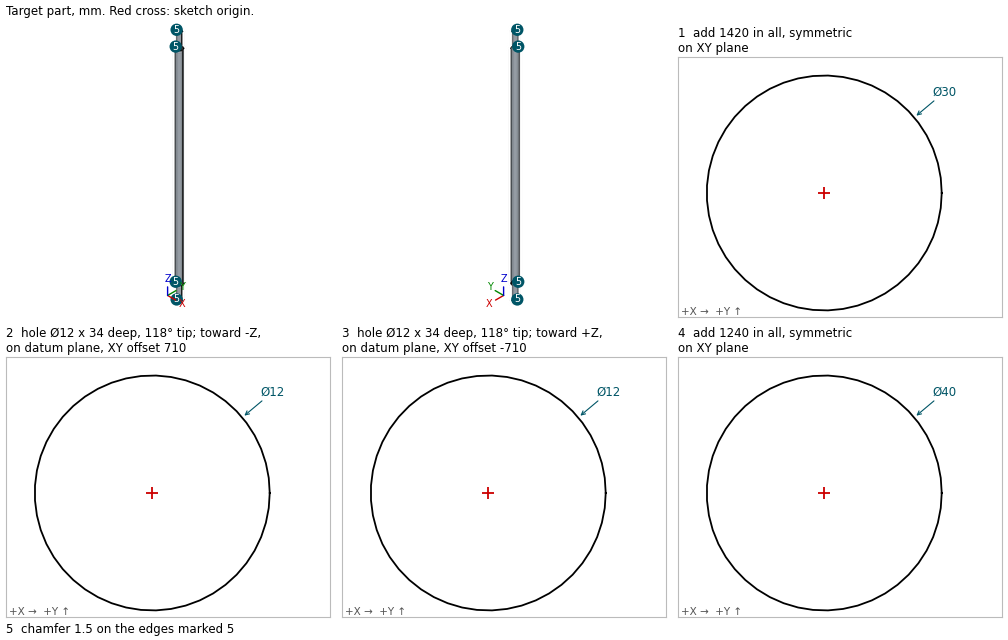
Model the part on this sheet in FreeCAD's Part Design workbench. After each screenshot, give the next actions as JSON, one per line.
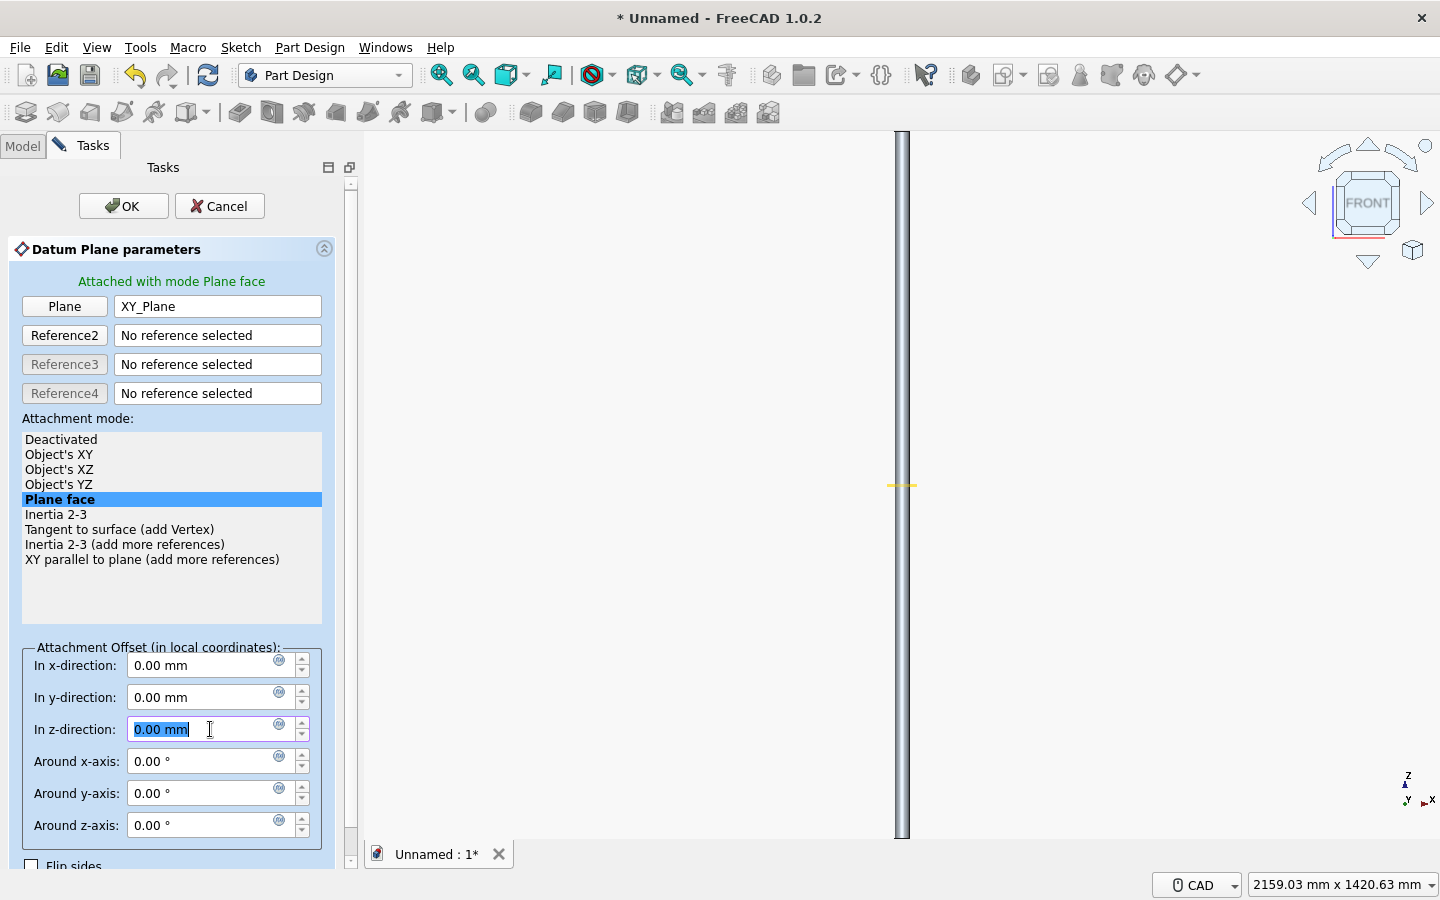
{"action": "type", "text": "710"}
{"action": "key", "text": "Tab"}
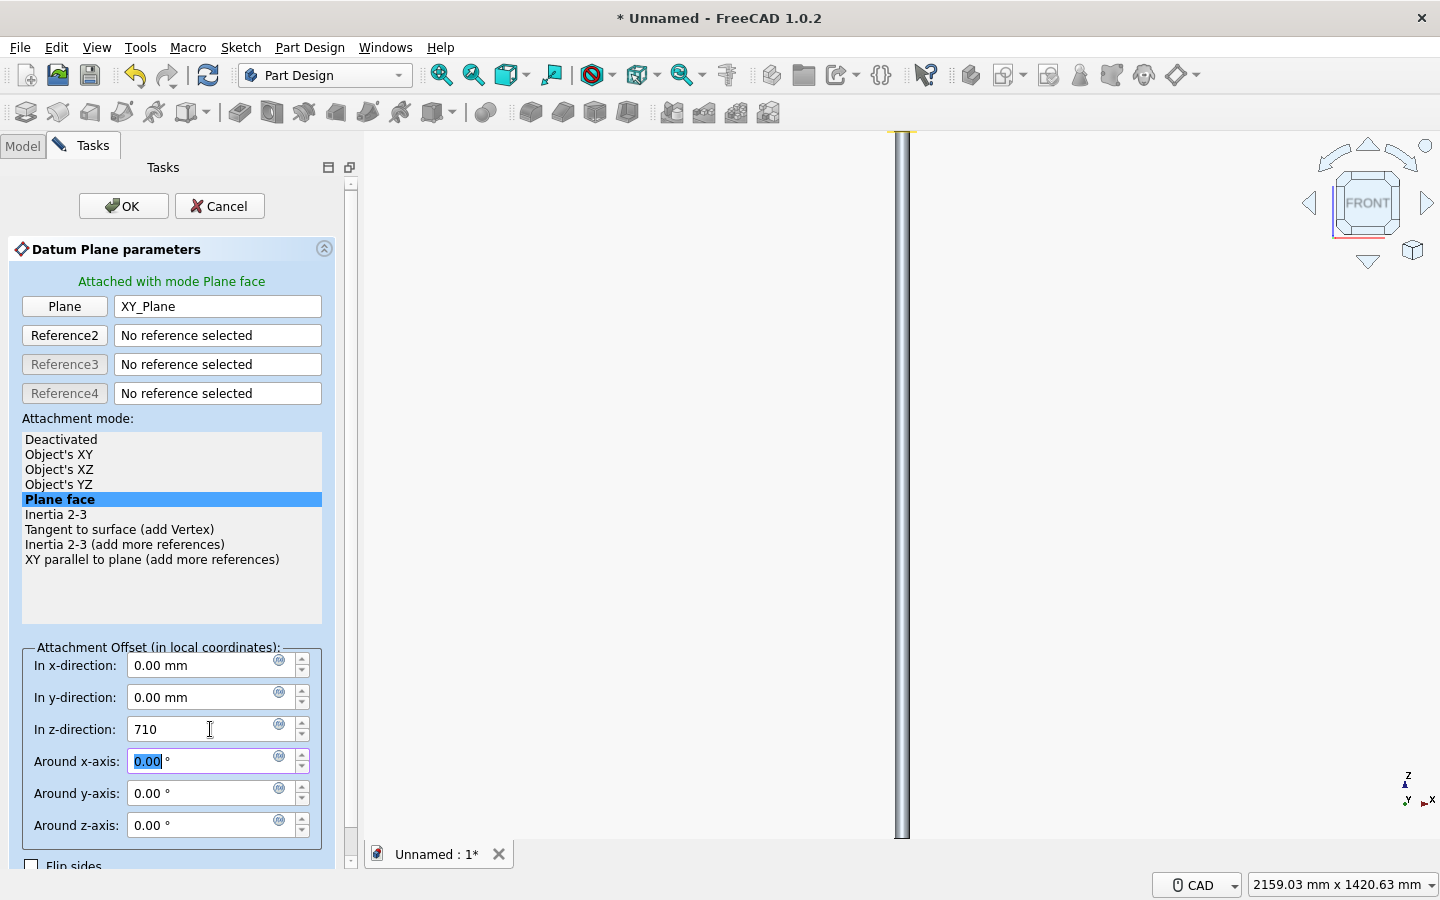
{"action": "left_click", "coordinate": [124, 206]}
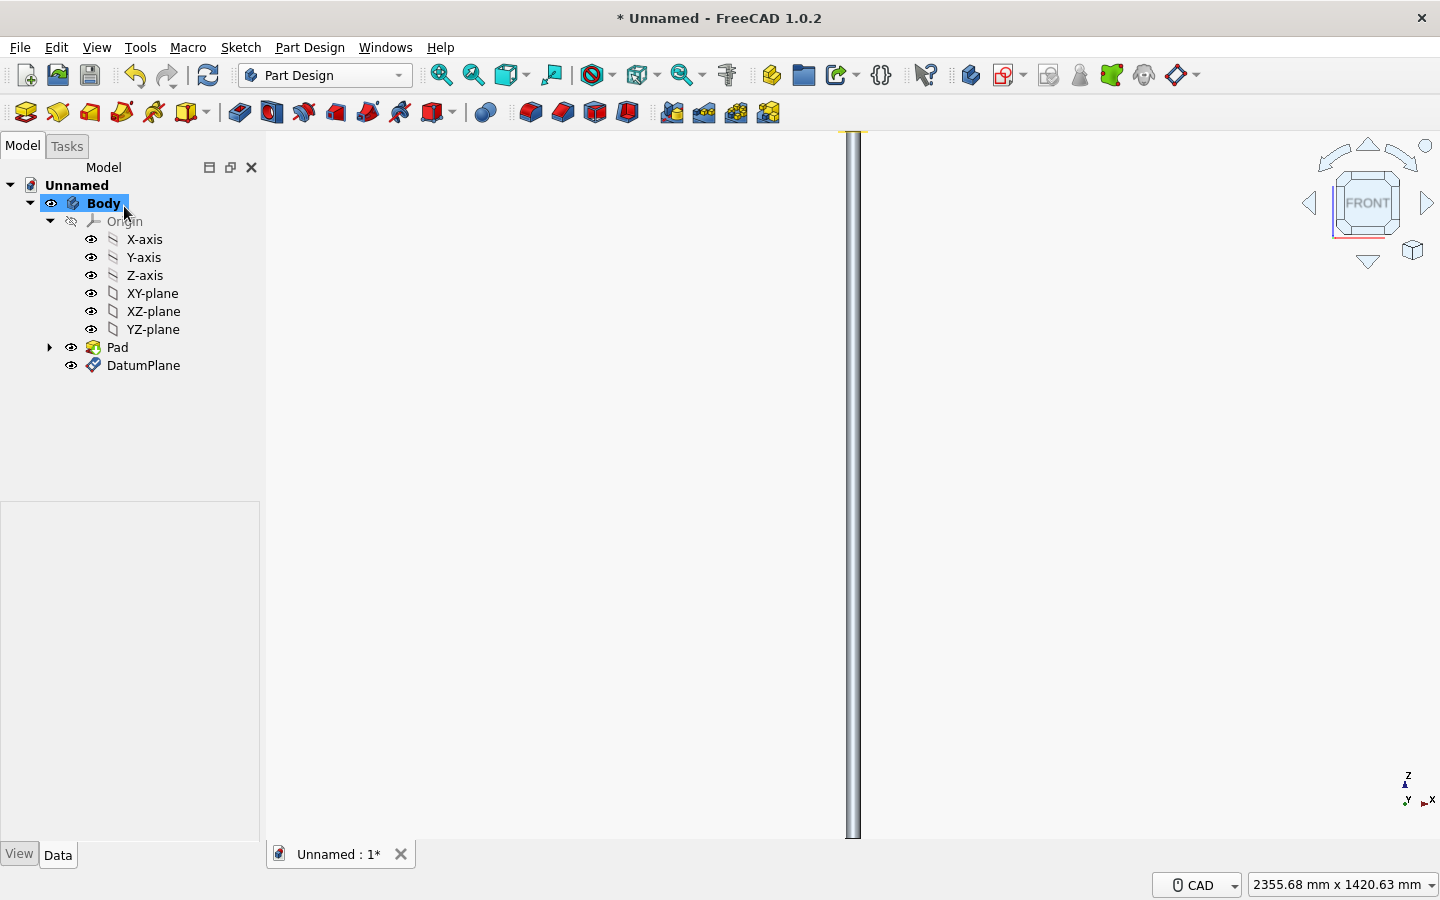
{"action": "left_click", "coordinate": [116, 365]}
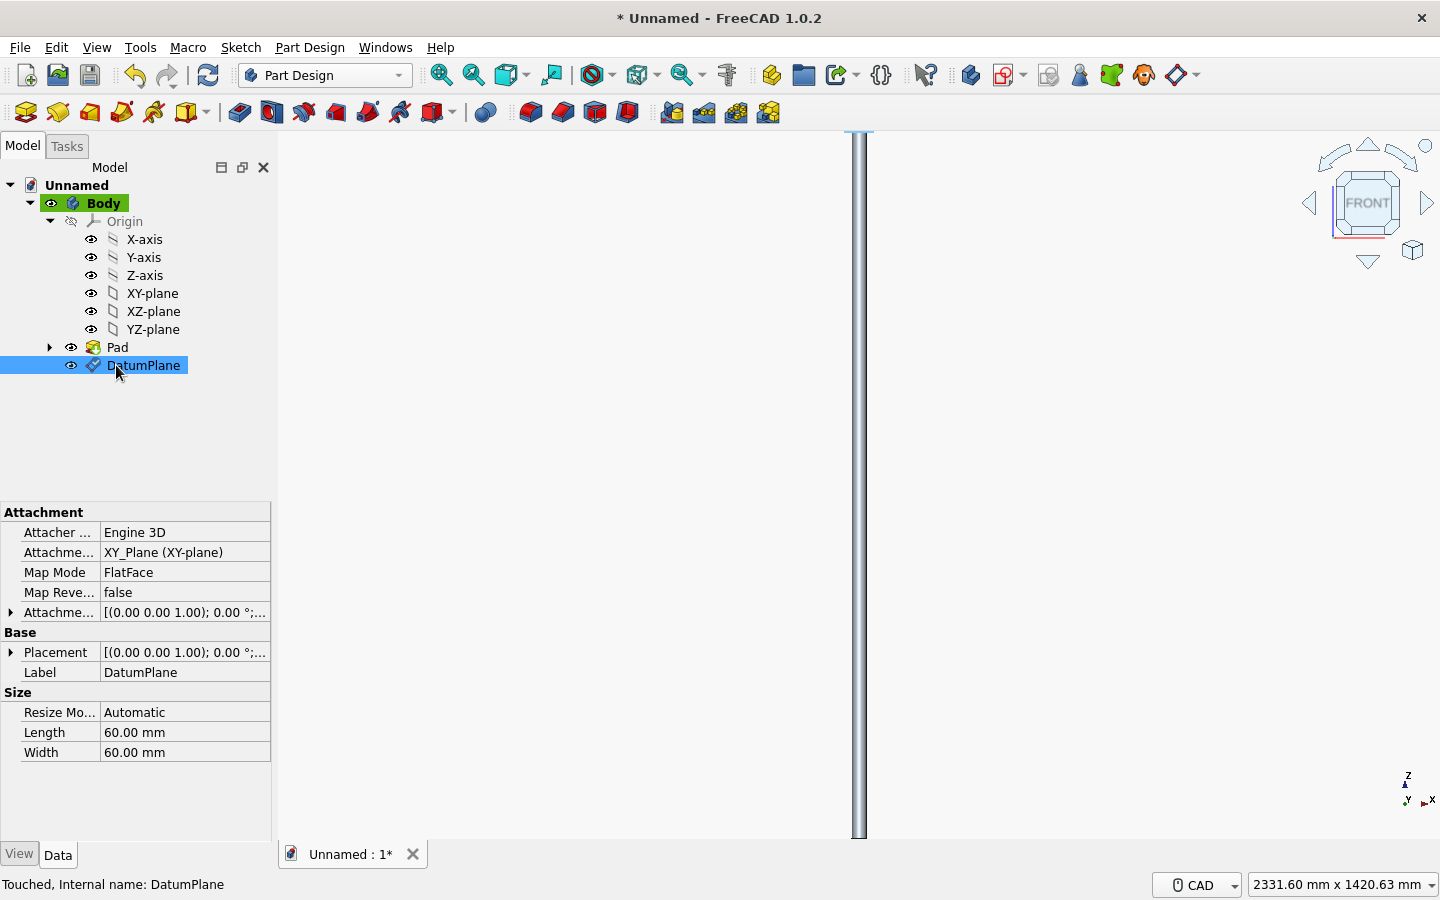
{"action": "left_click", "coordinate": [1004, 76]}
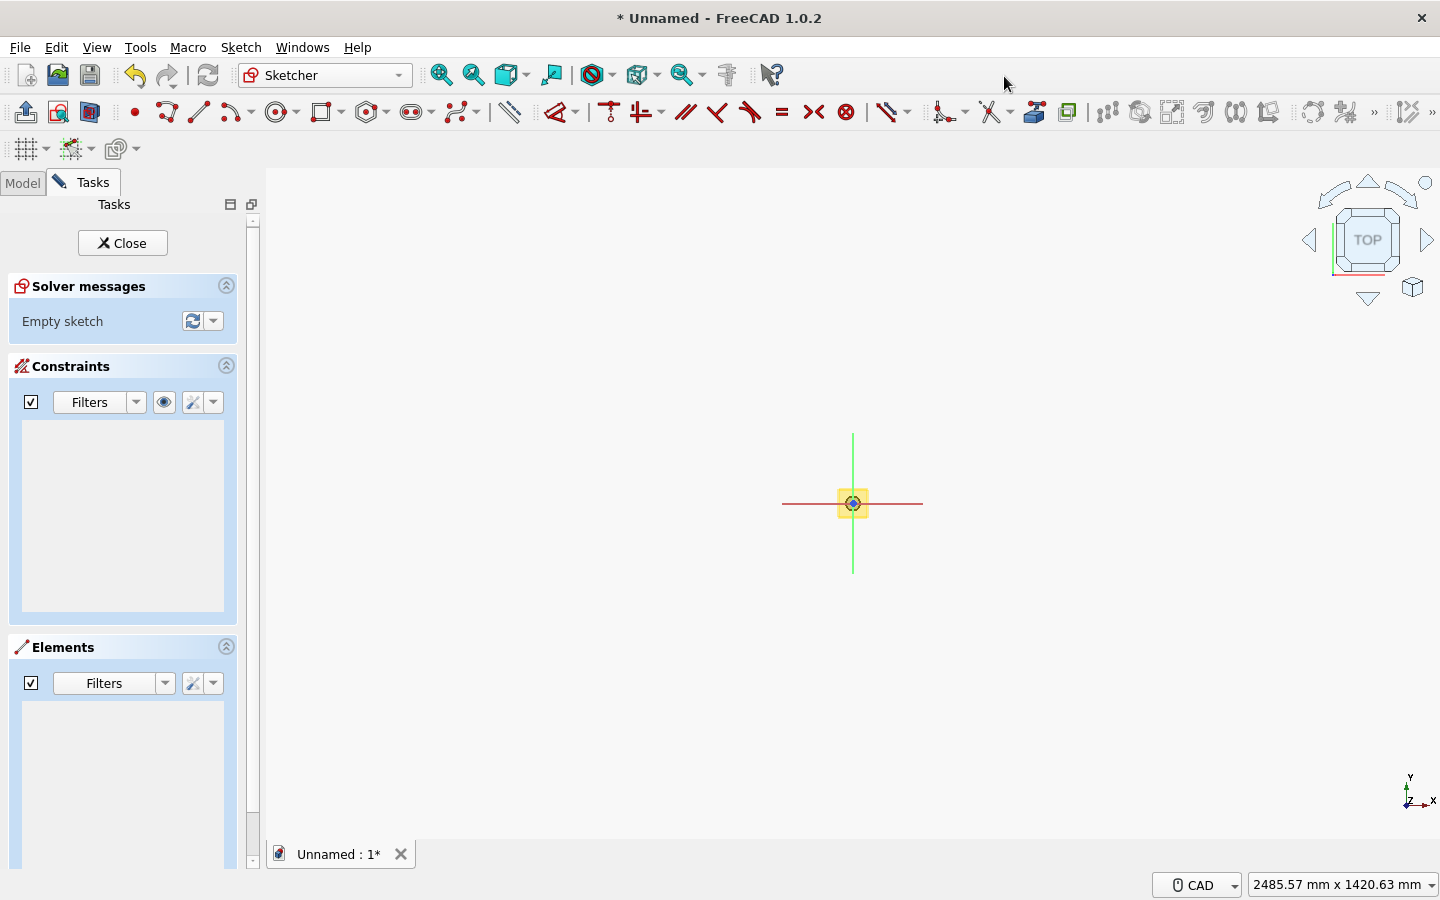
{"action": "scroll", "coordinate": [857, 504], "scroll_direction": "up", "scroll_amount": 15}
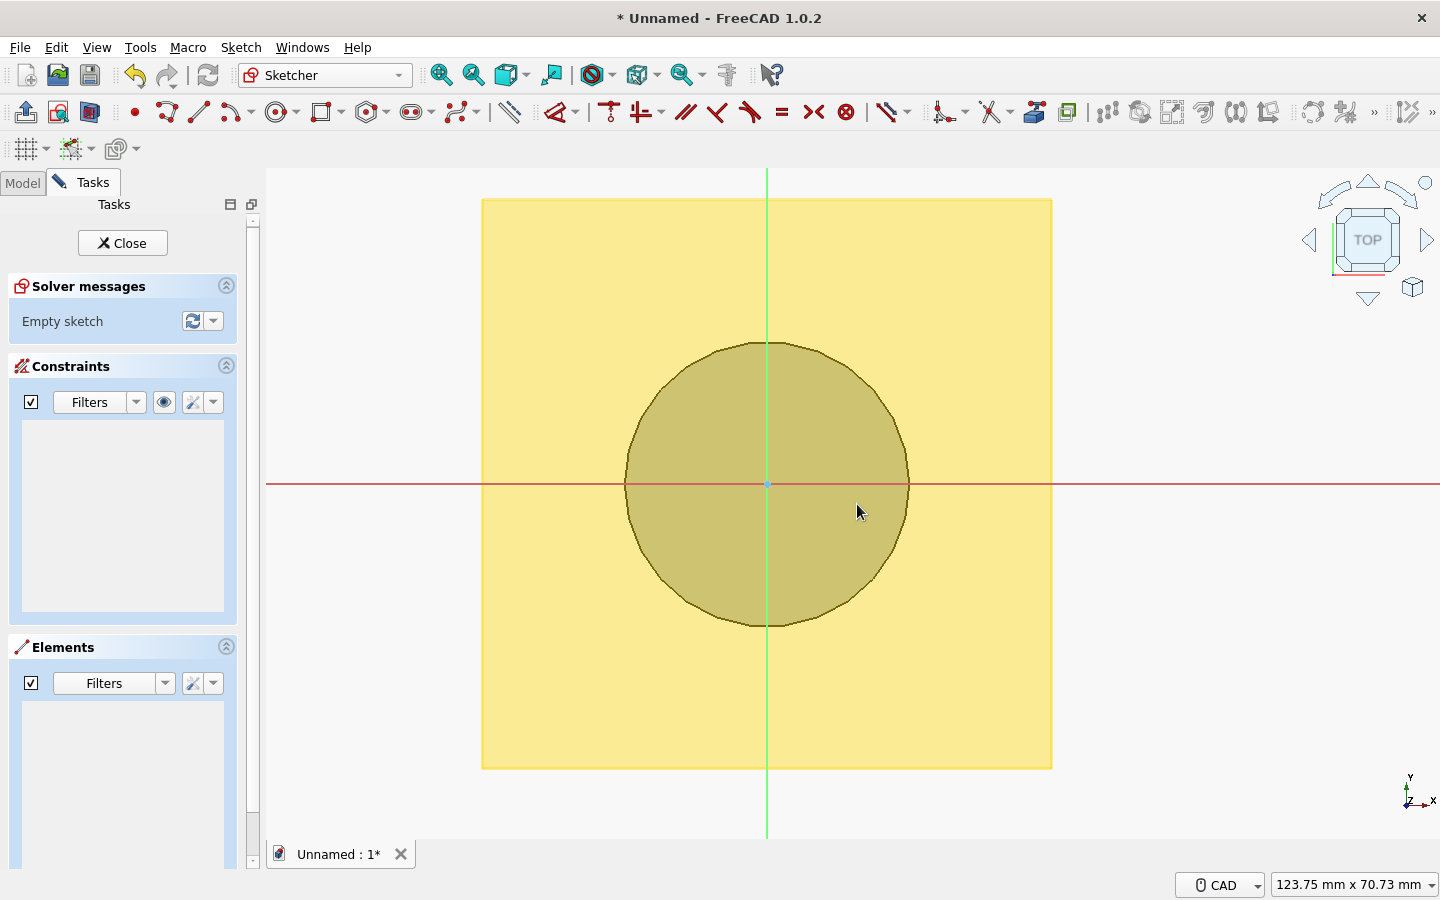
{"action": "scroll", "coordinate": [761, 478], "scroll_direction": "up", "scroll_amount": 7}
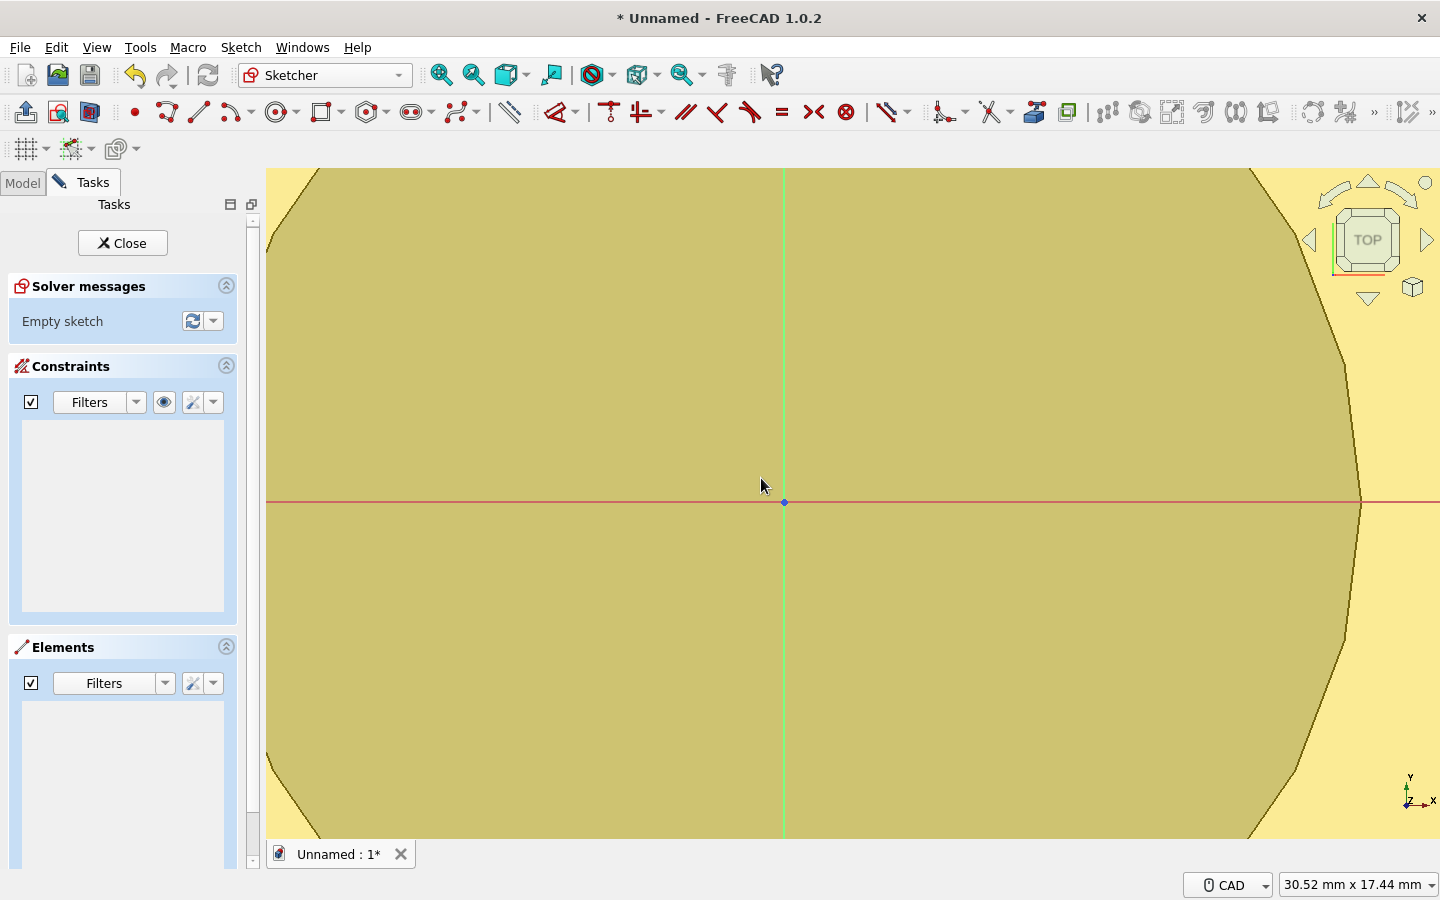
{"action": "left_click", "coordinate": [276, 112]}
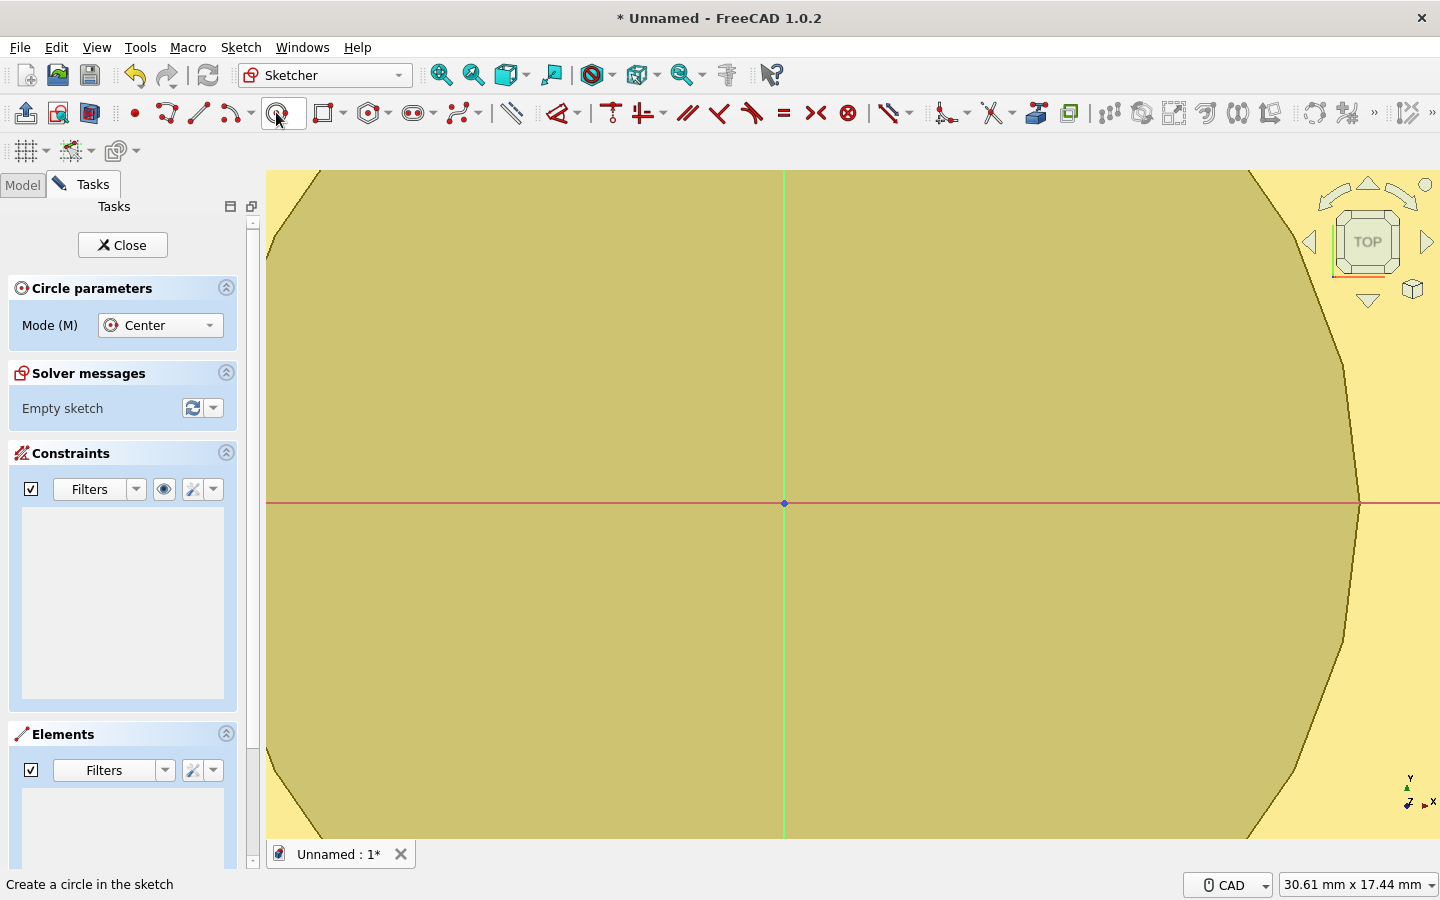
{"action": "left_click", "coordinate": [784, 503]}
{"action": "mouse_move", "coordinate": [947, 341]}